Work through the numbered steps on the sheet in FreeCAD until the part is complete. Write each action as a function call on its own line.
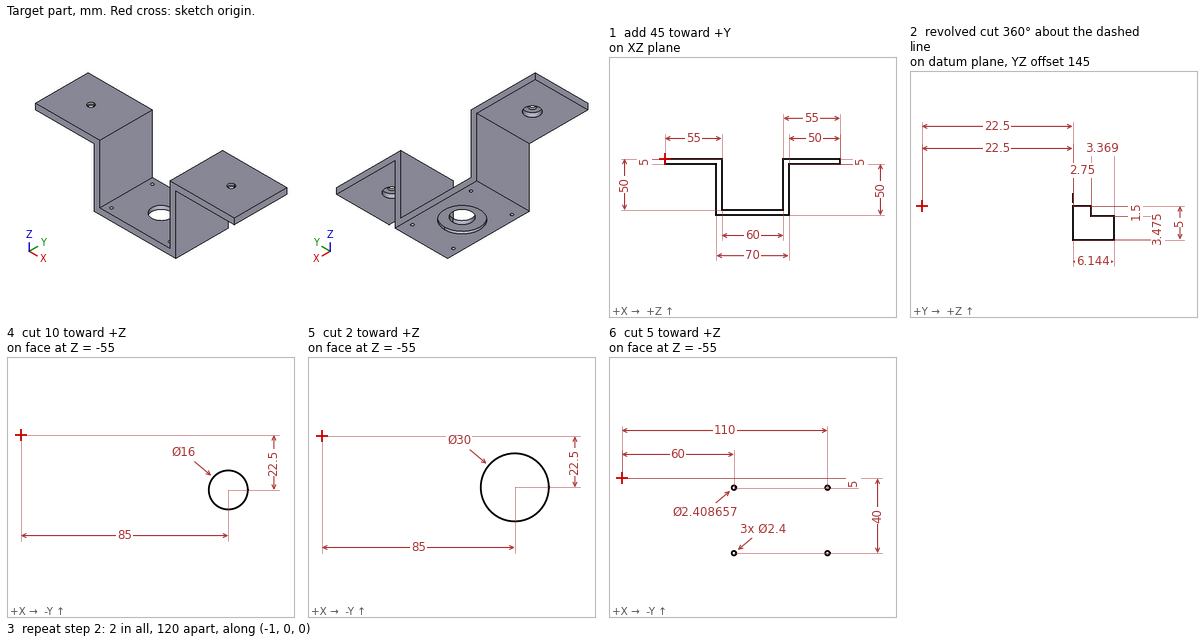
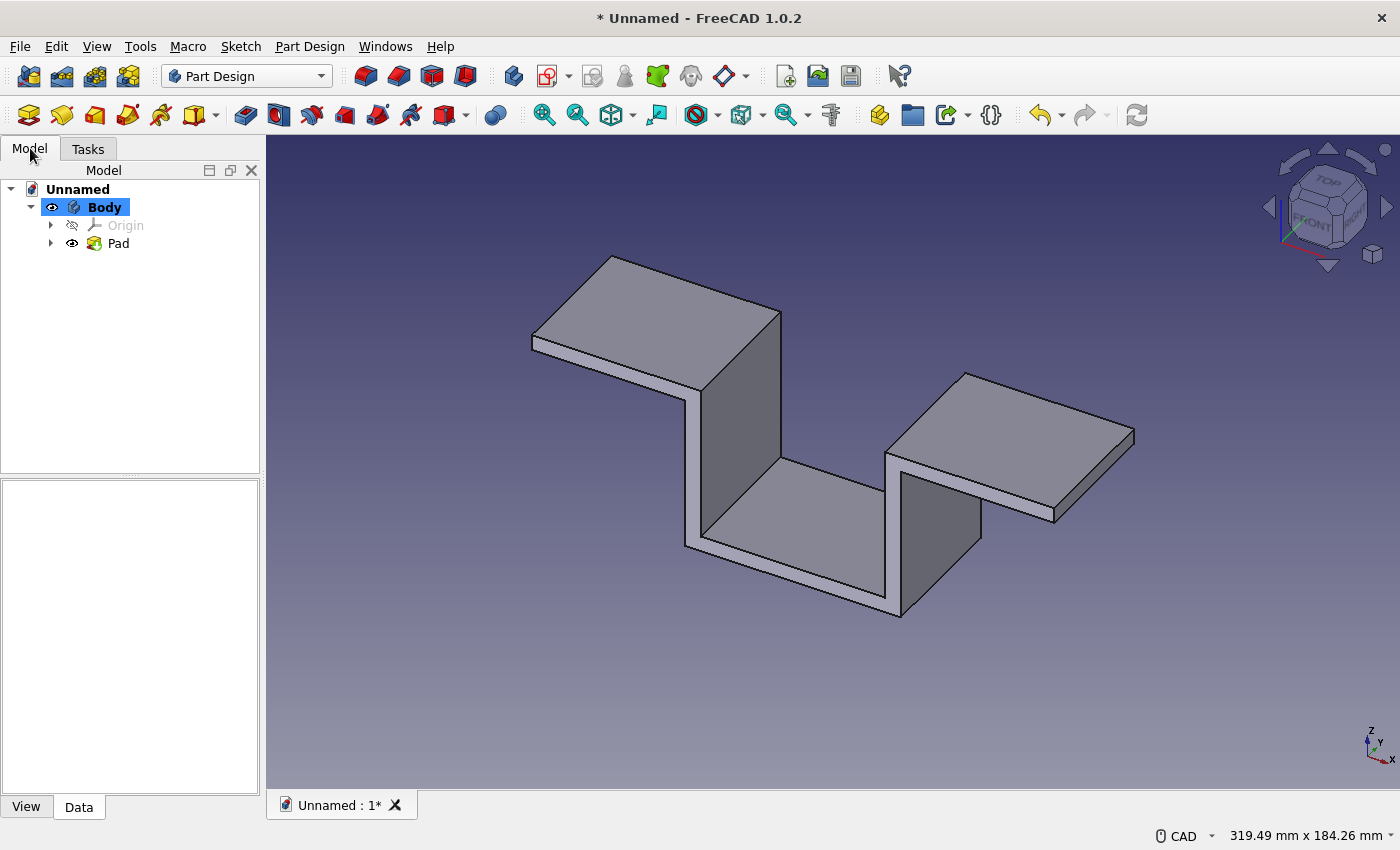
click(51, 225)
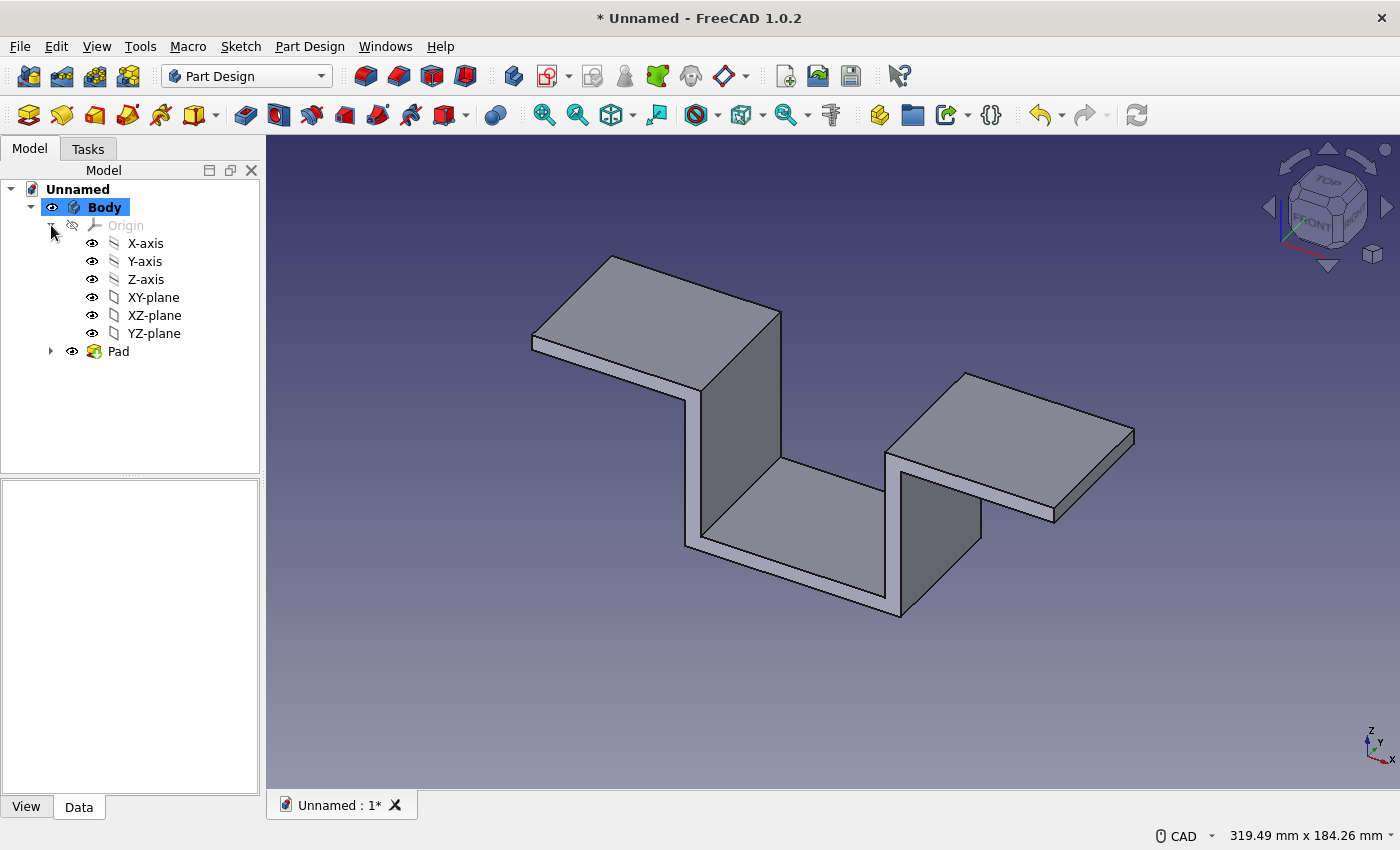
click(137, 333)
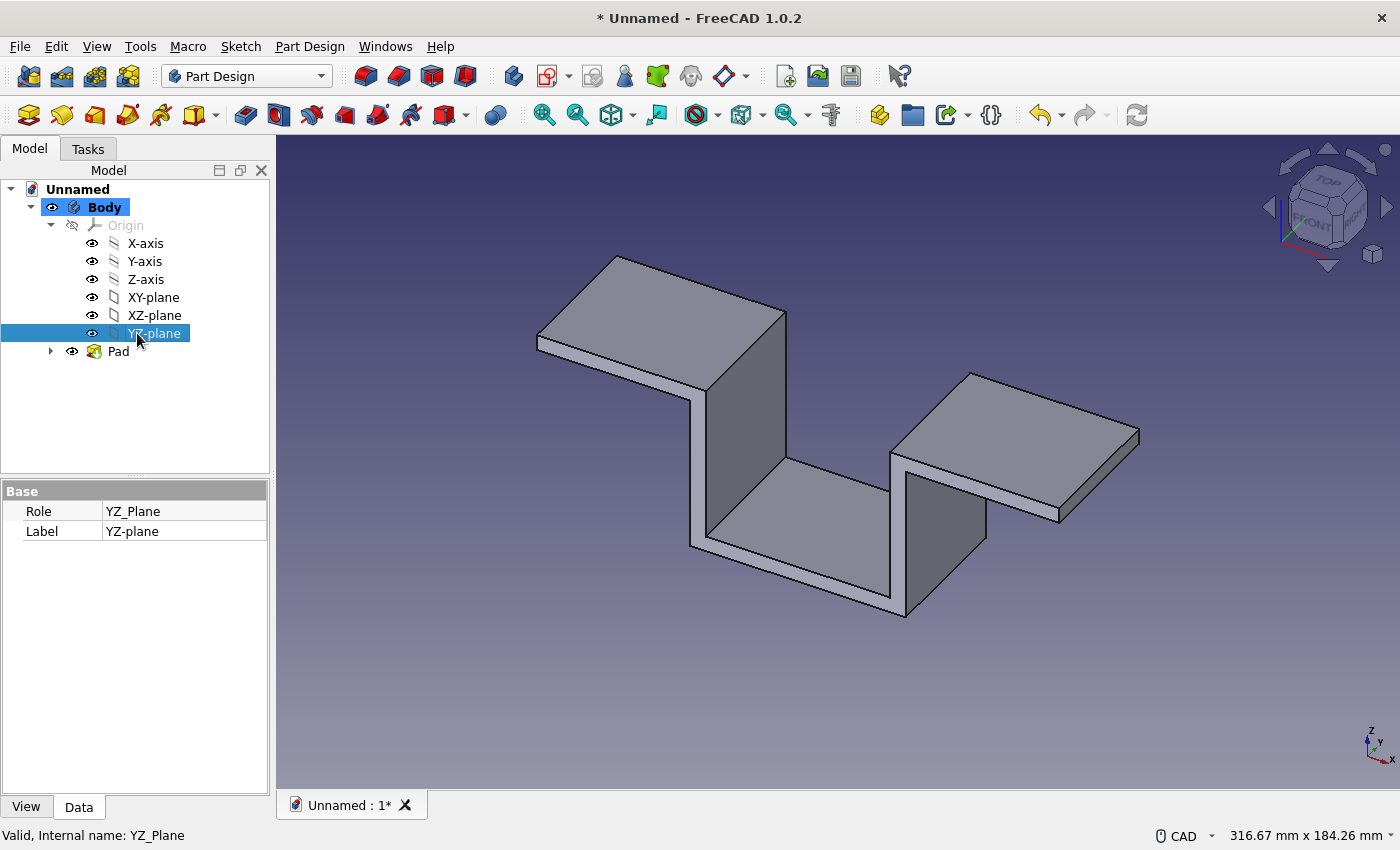
click(724, 76)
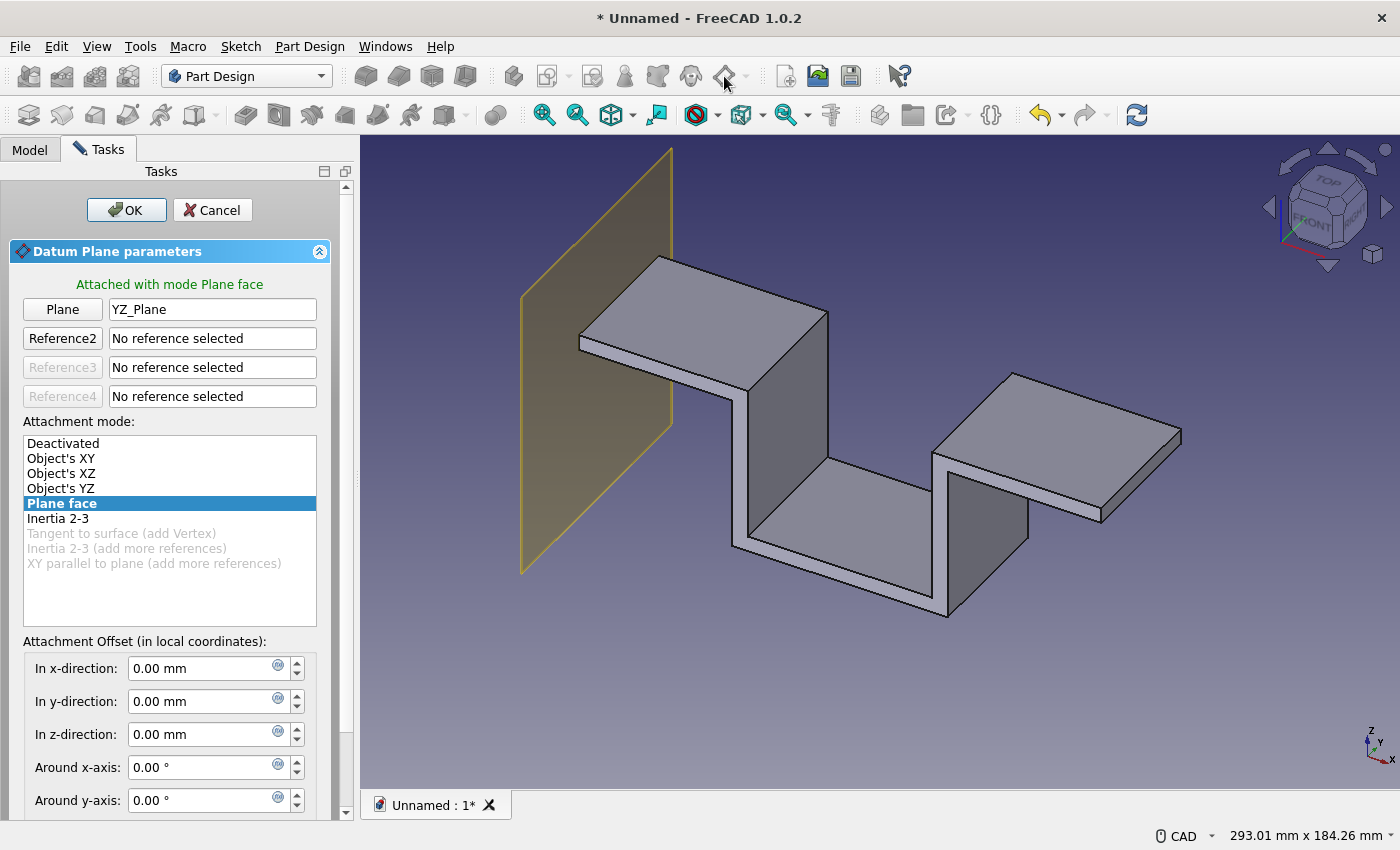
triple_click(210, 734)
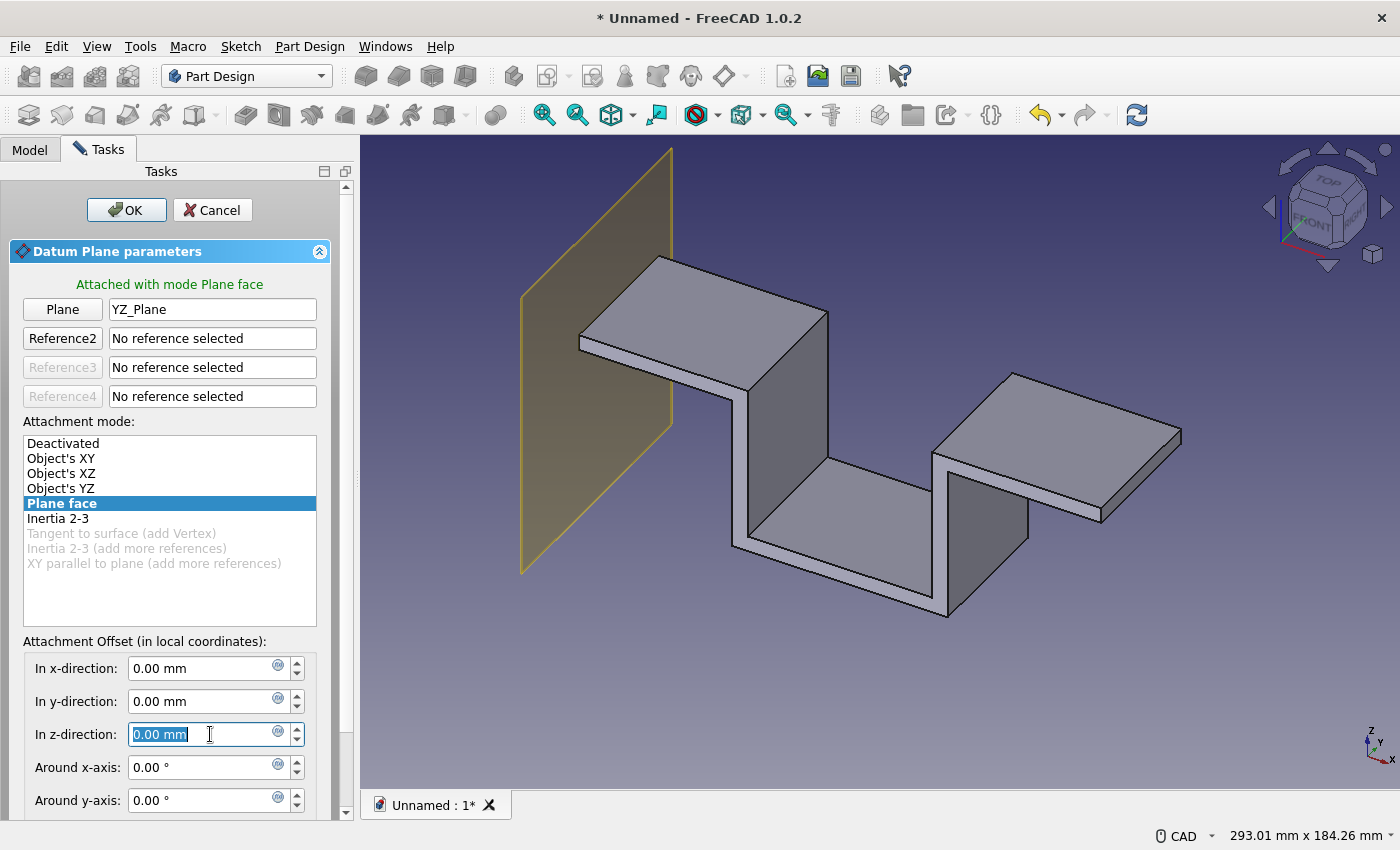
text(145)
key(Tab)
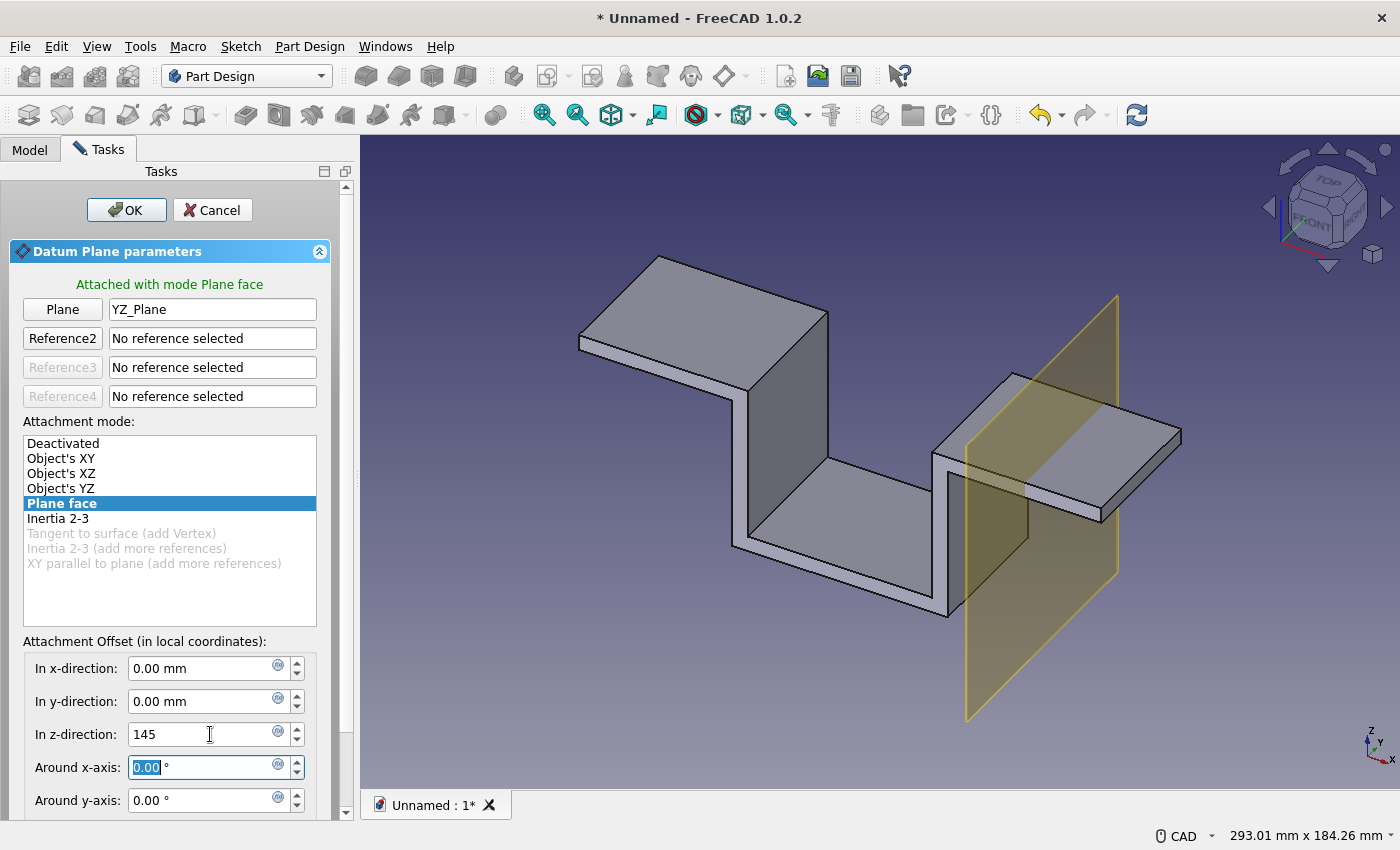
click(127, 210)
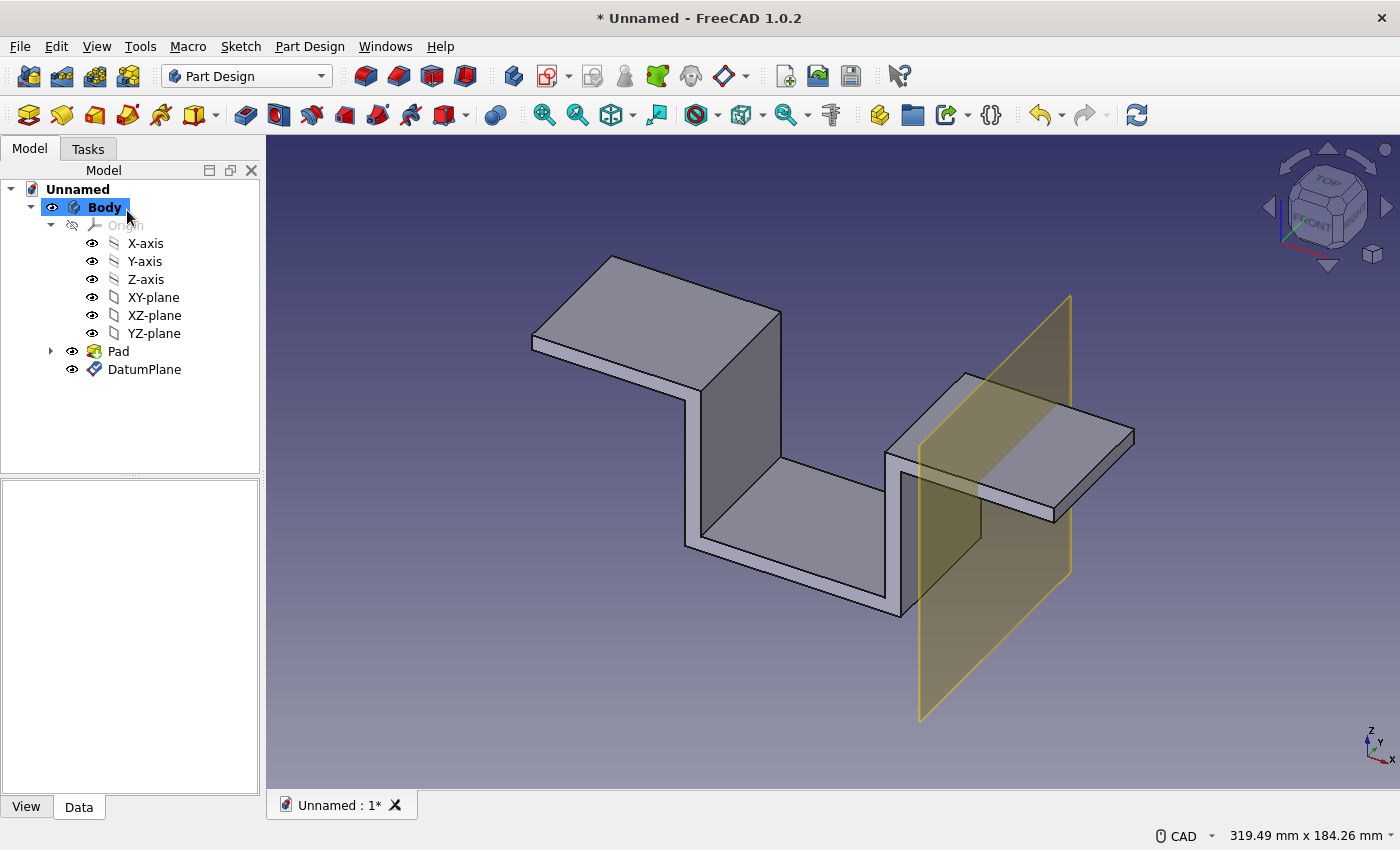
click(117, 369)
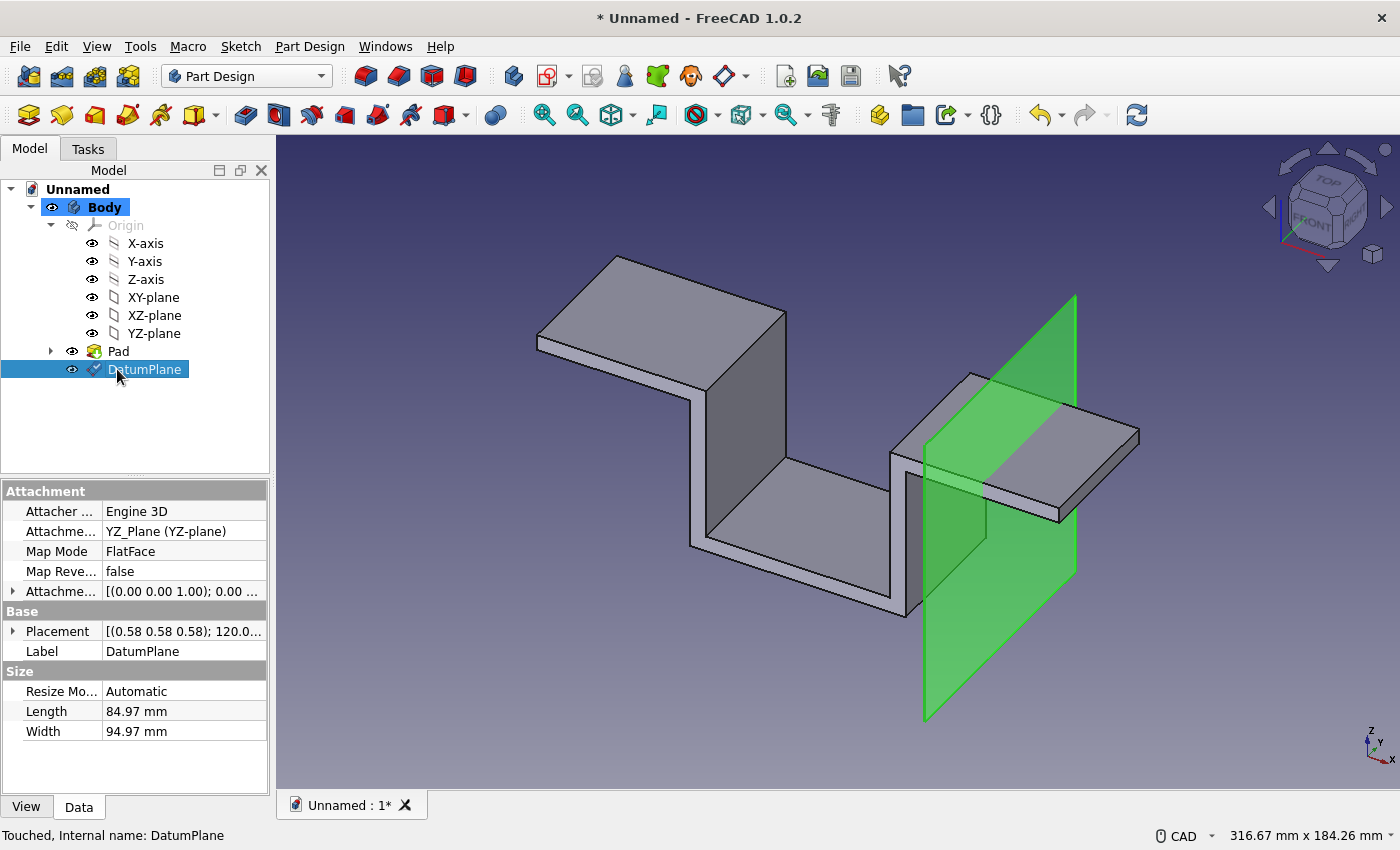
click(546, 76)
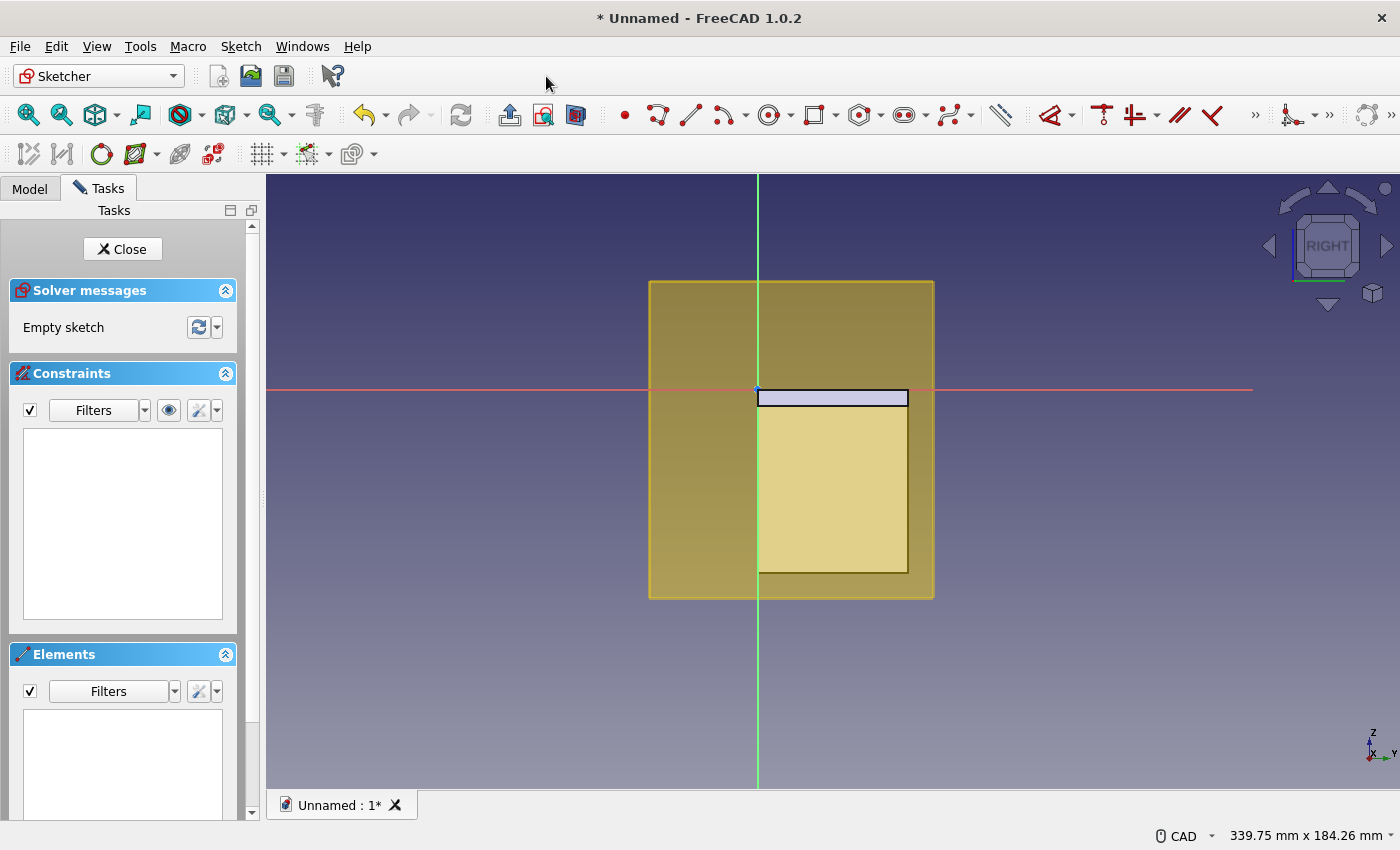
click(576, 116)